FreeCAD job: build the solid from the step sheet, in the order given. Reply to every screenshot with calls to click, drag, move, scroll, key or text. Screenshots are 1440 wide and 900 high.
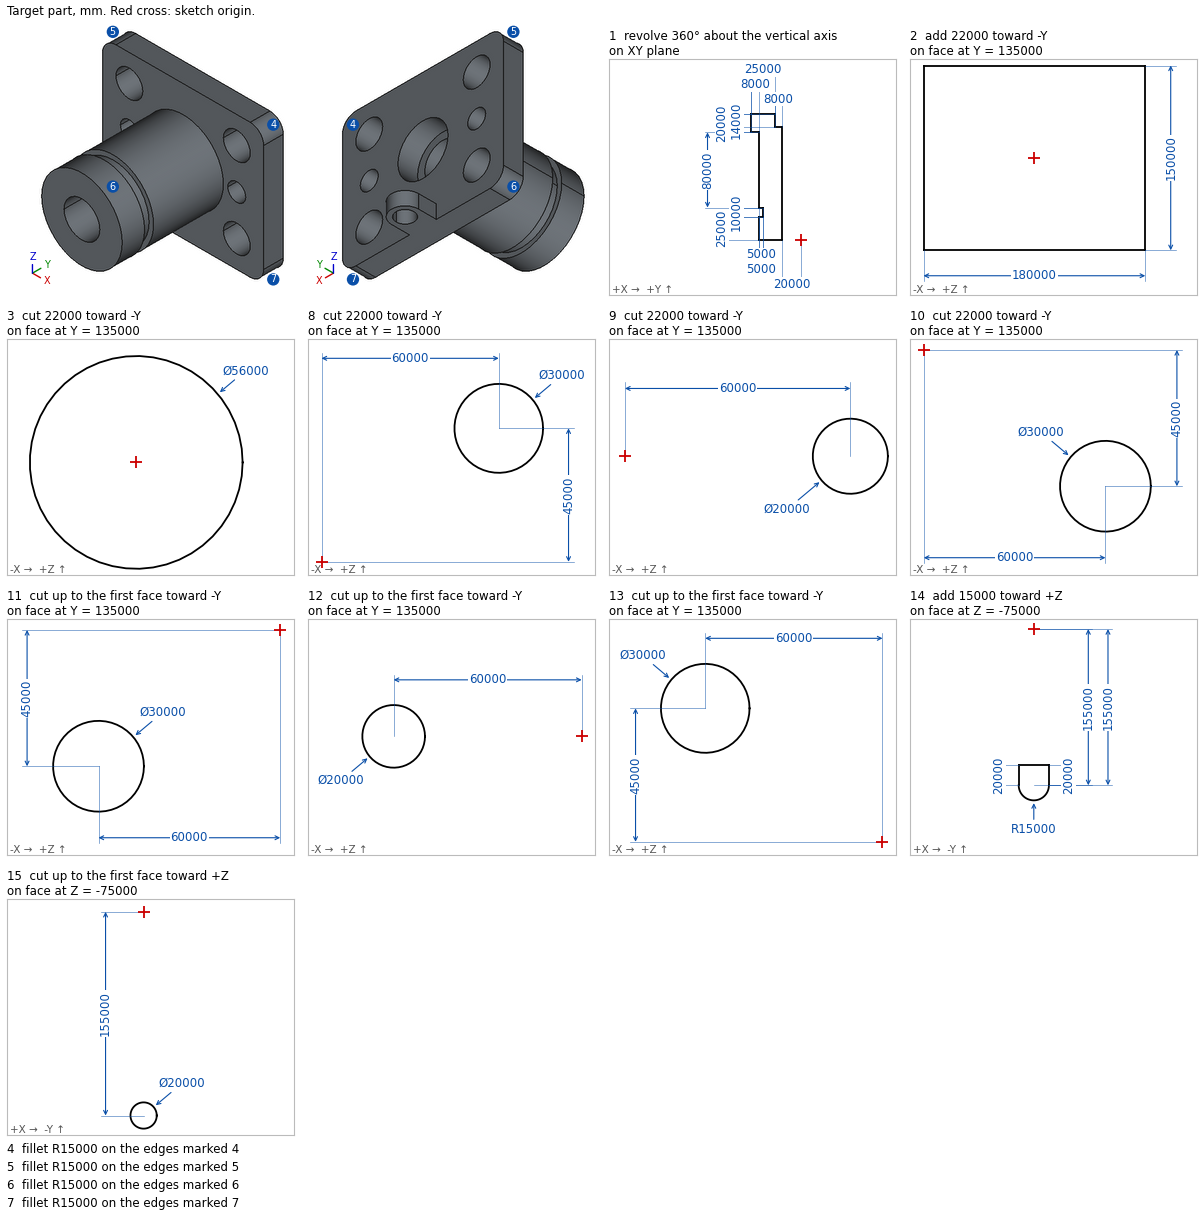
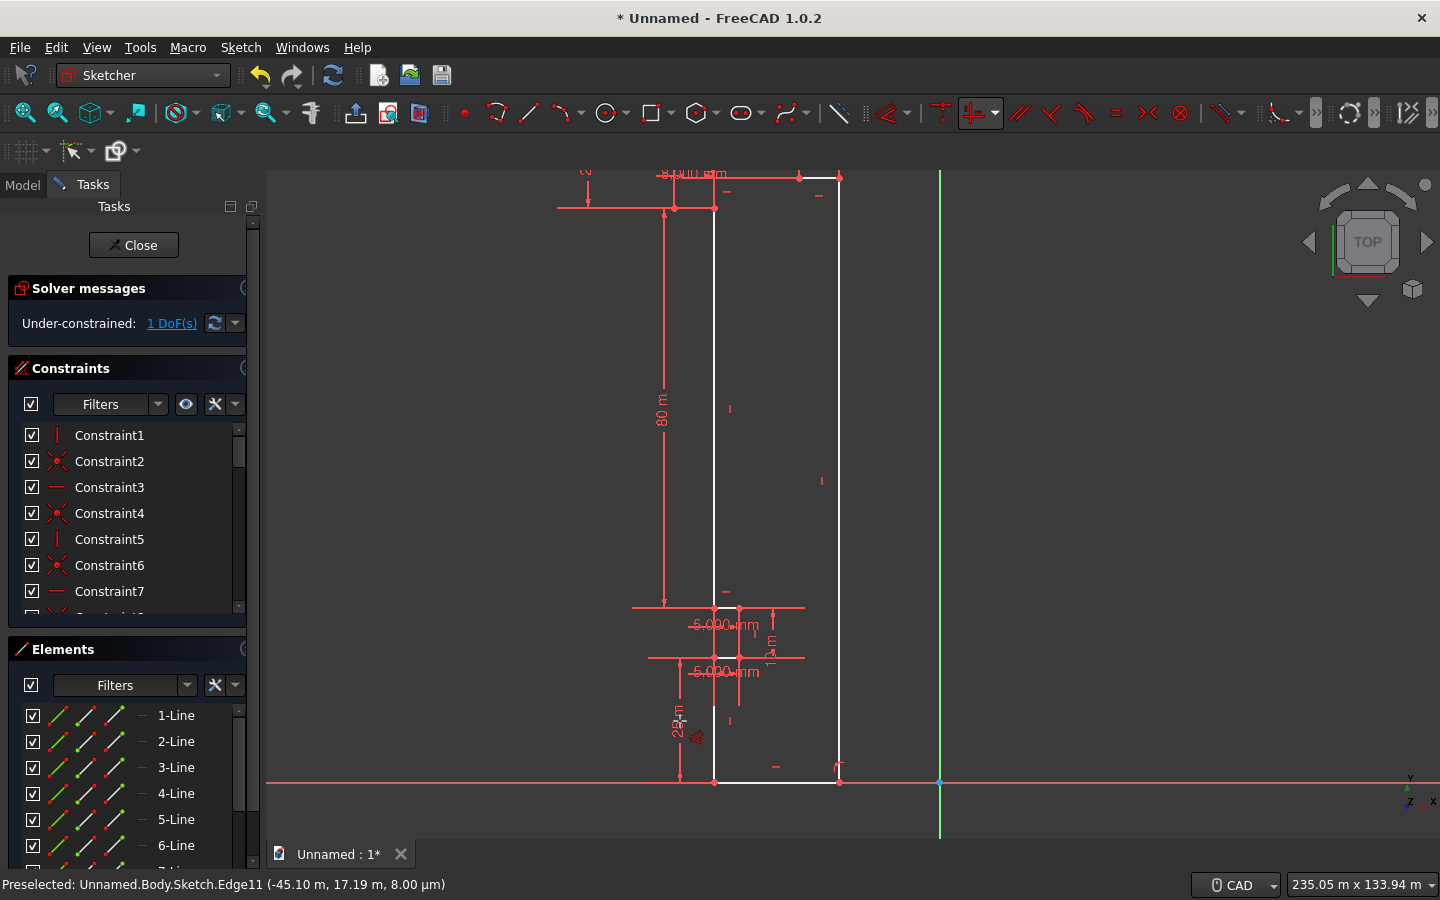
click(839, 783)
click(889, 749)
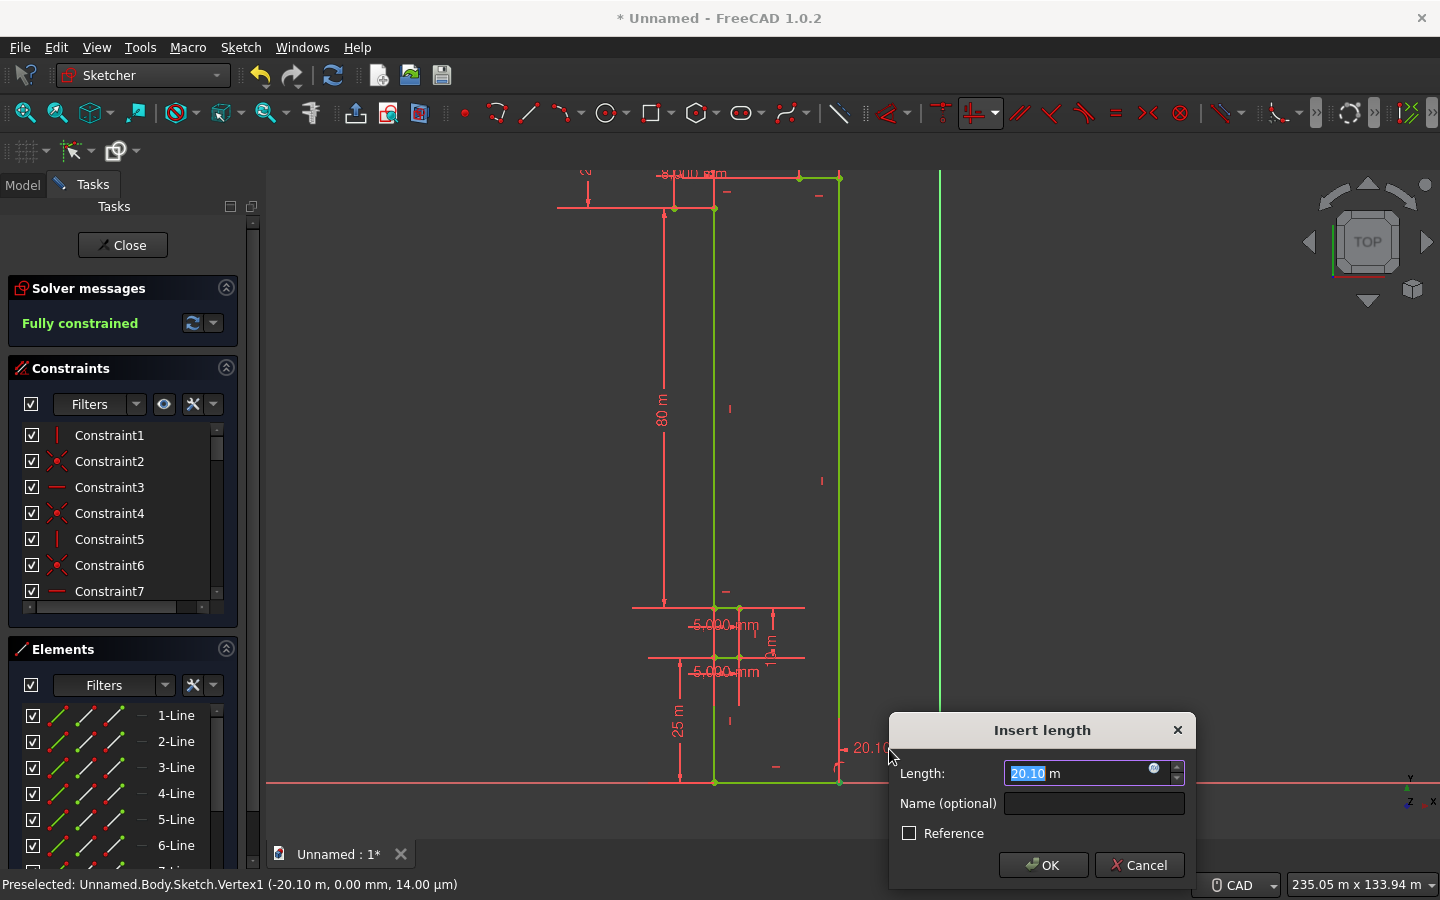
key(ctrl+a)
text(20000 mm)
key(Return)
key(Escape)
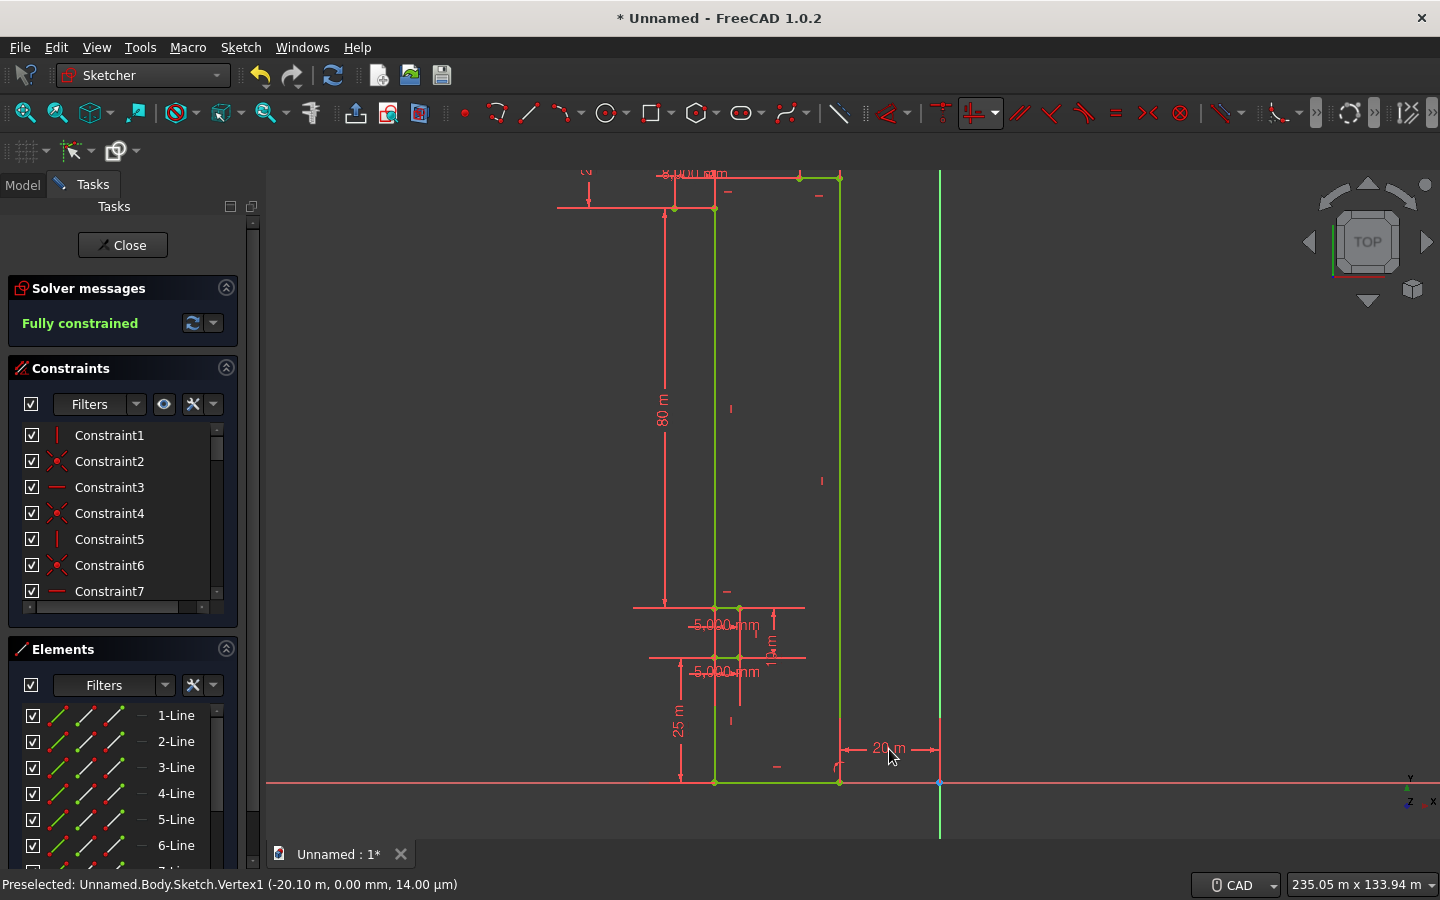
click(123, 245)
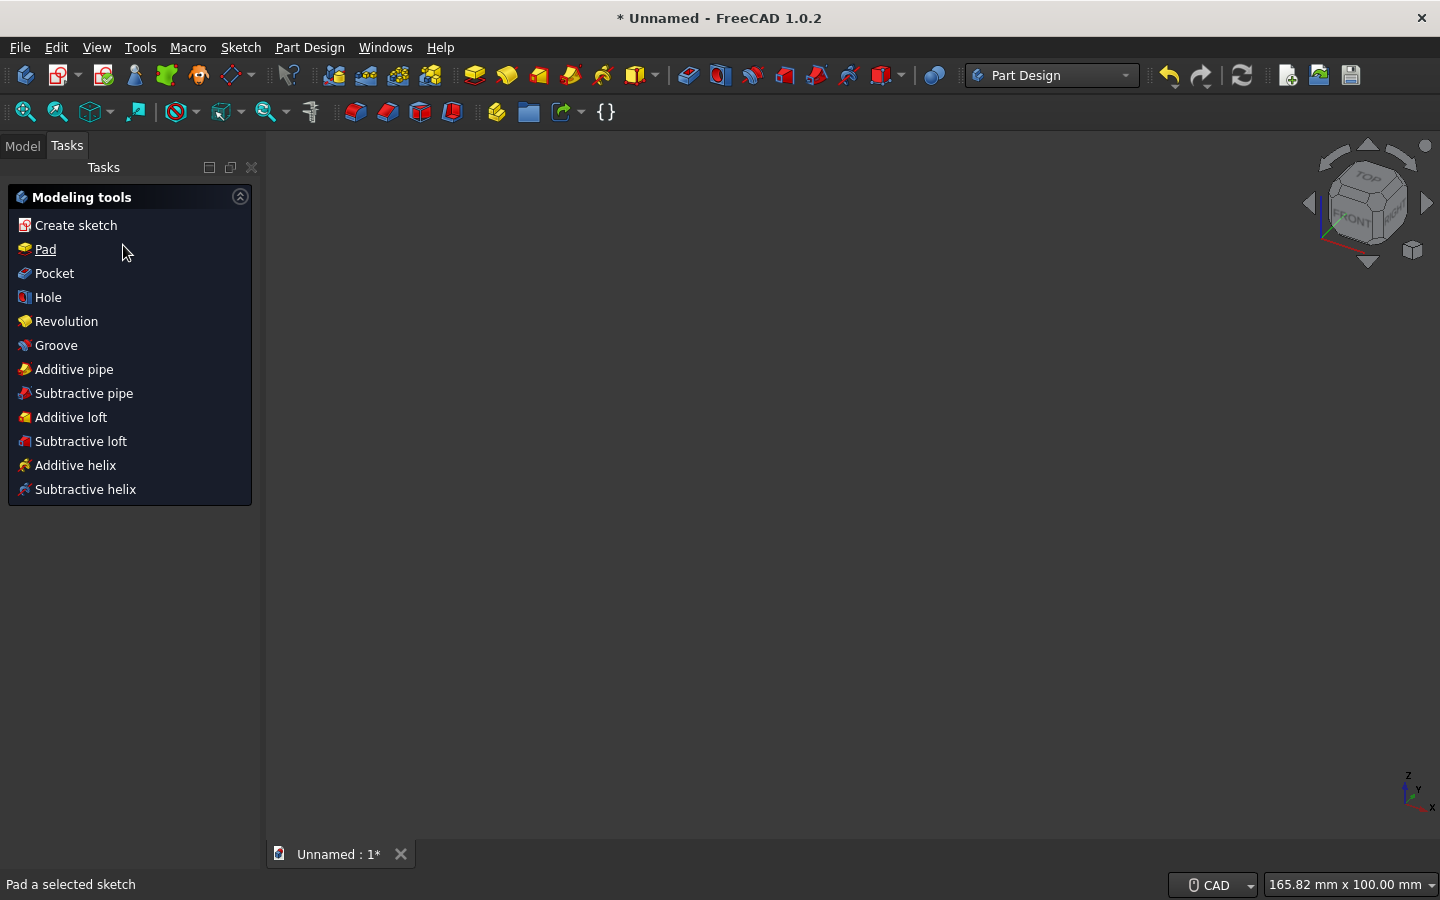
click(508, 76)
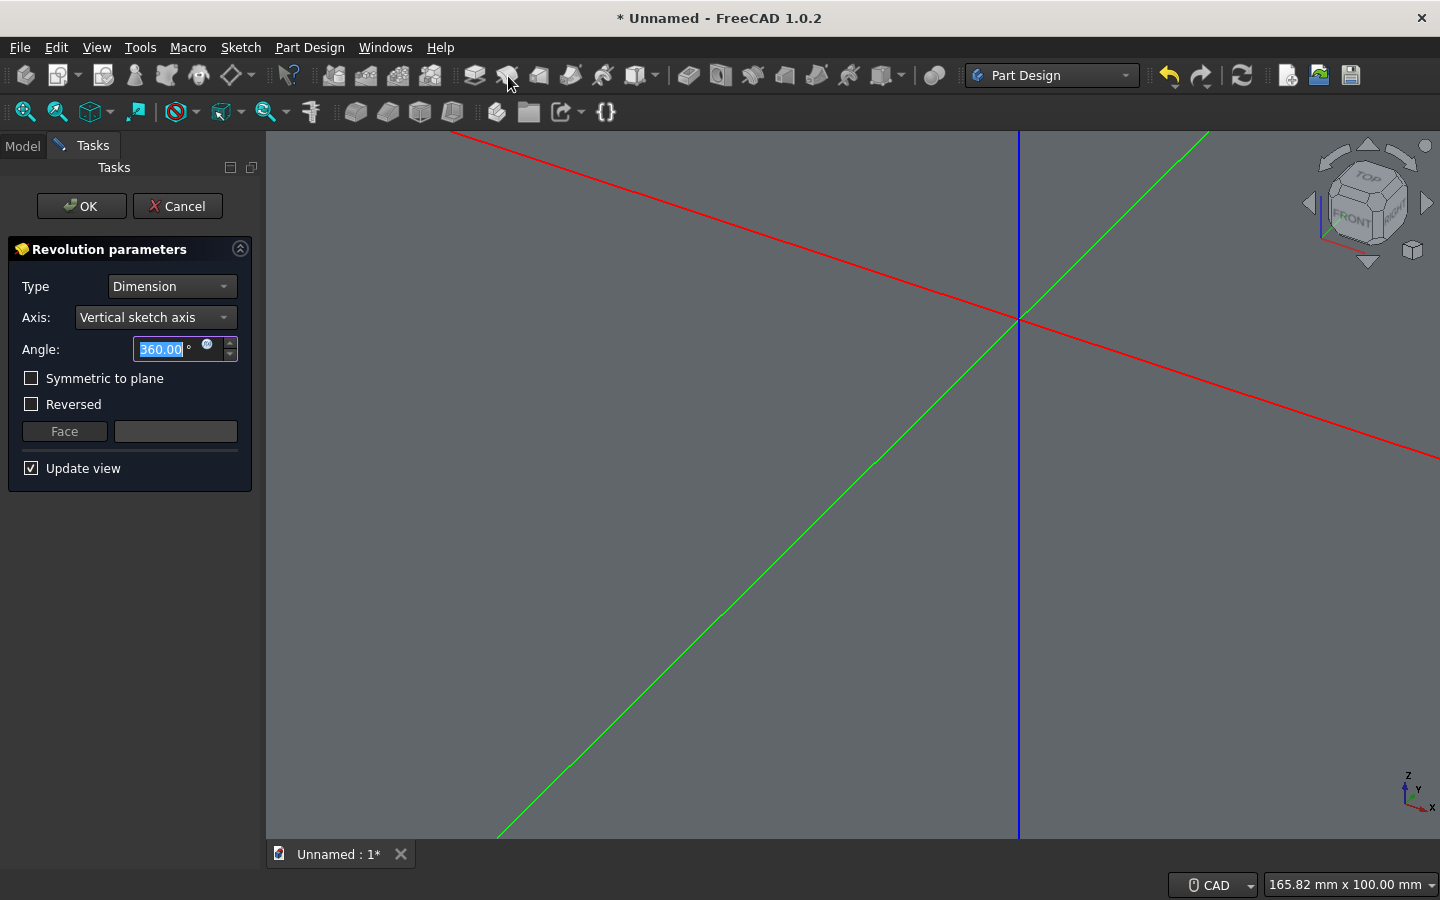
click(82, 206)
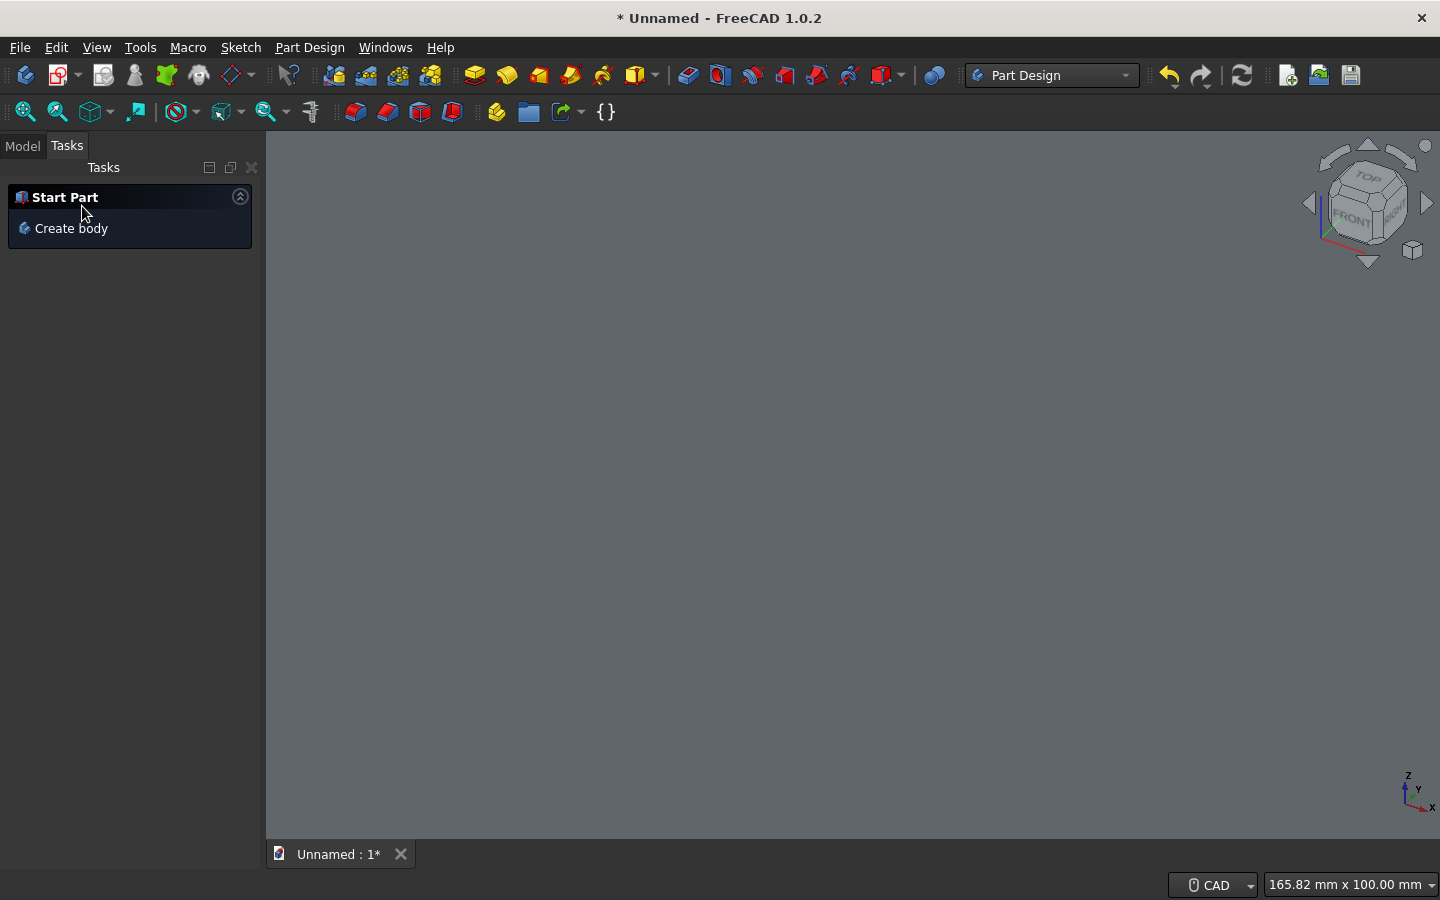
click(26, 112)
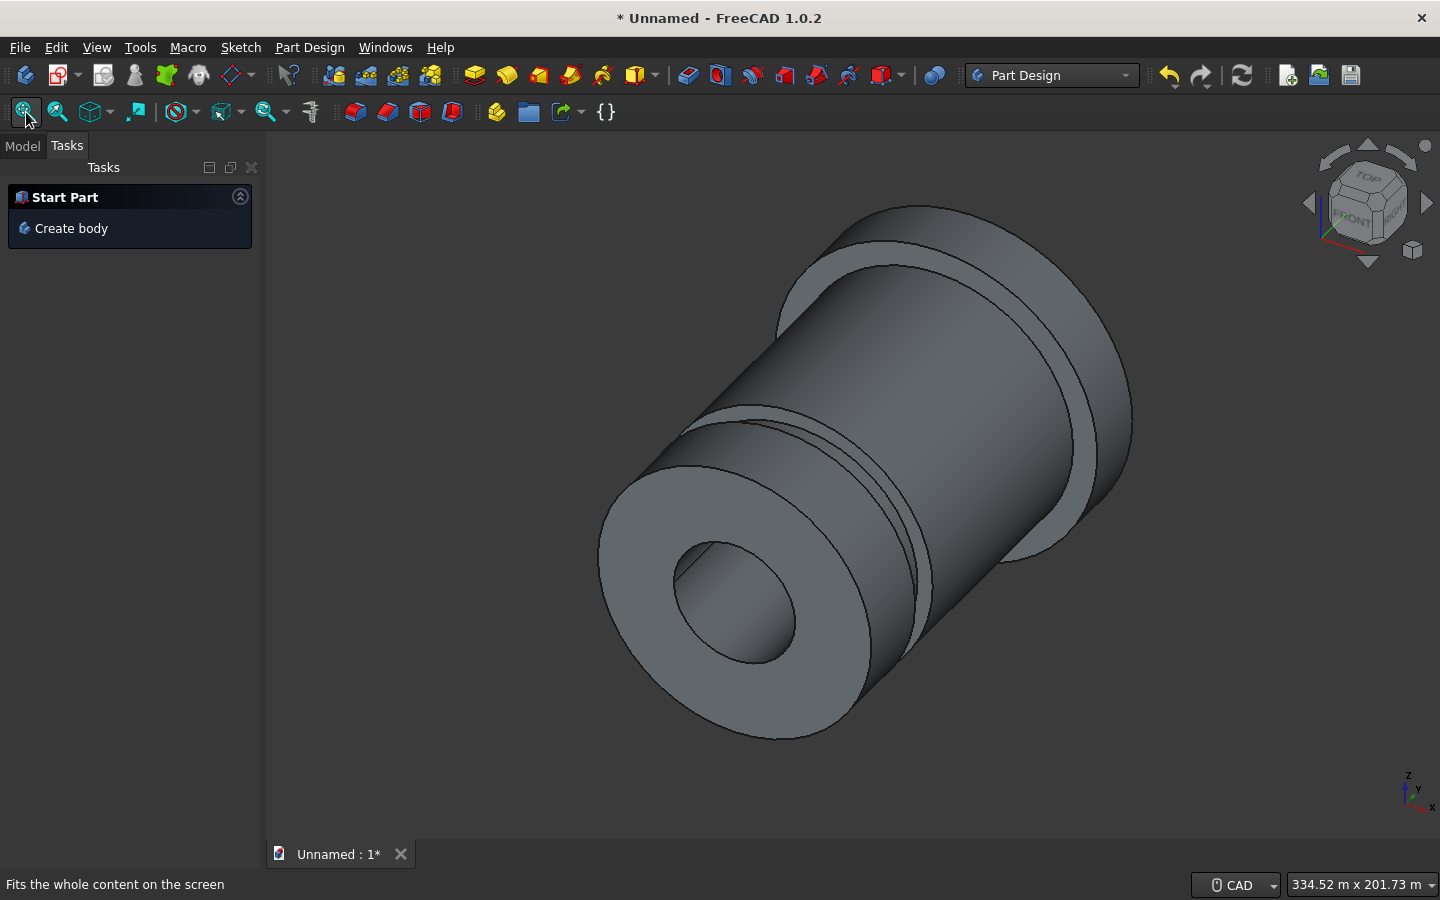
key(4)